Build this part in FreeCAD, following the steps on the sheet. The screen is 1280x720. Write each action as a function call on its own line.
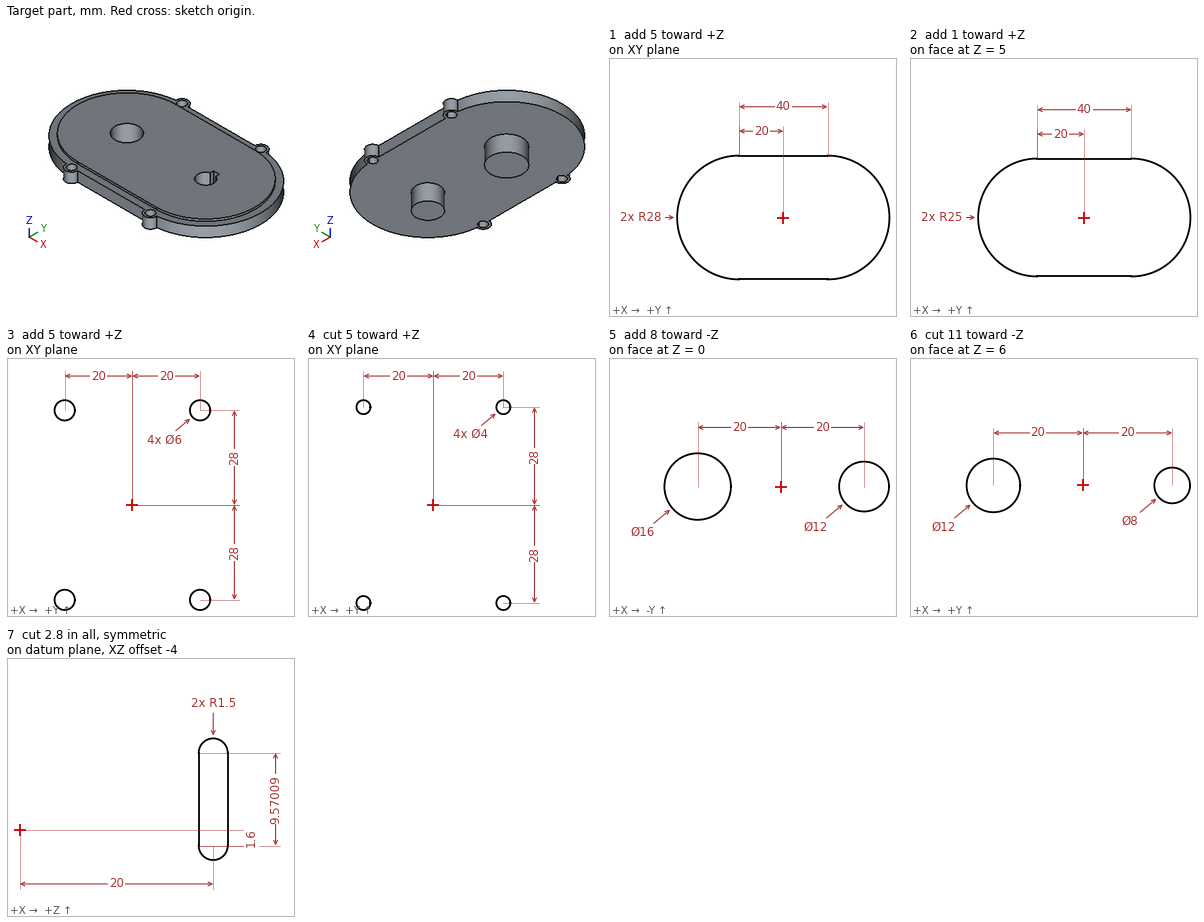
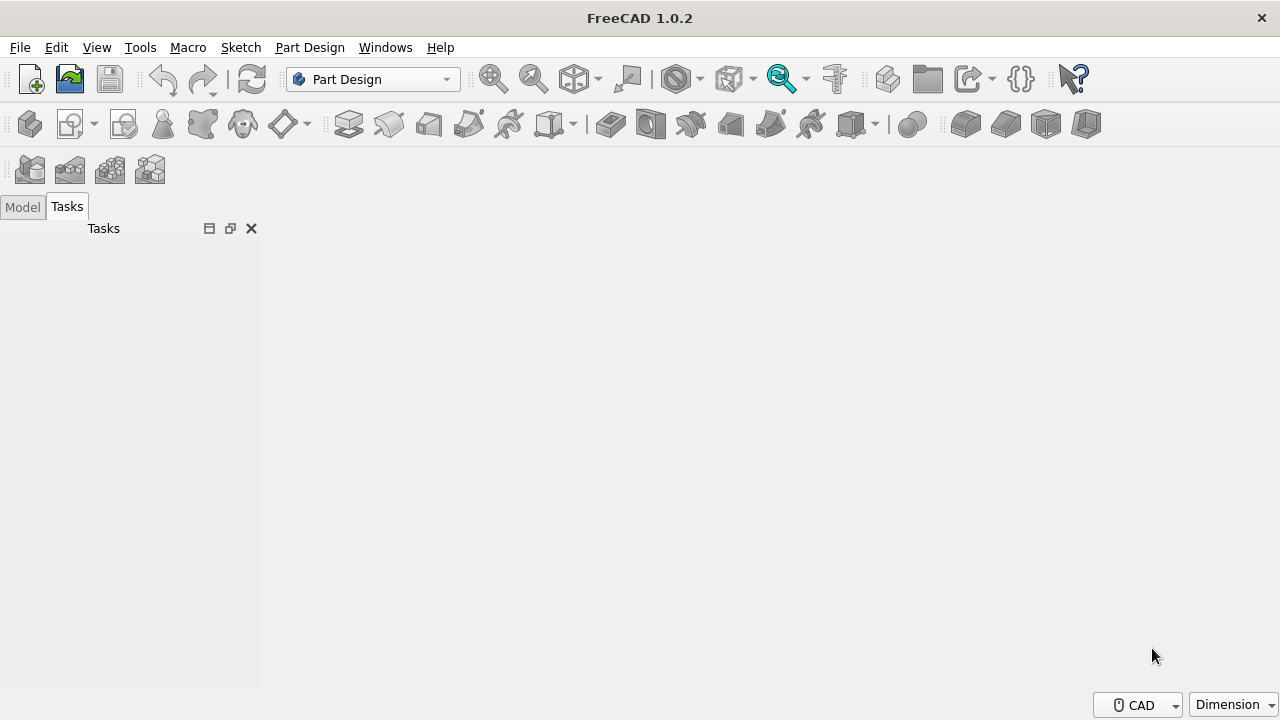
key(ctrl+n)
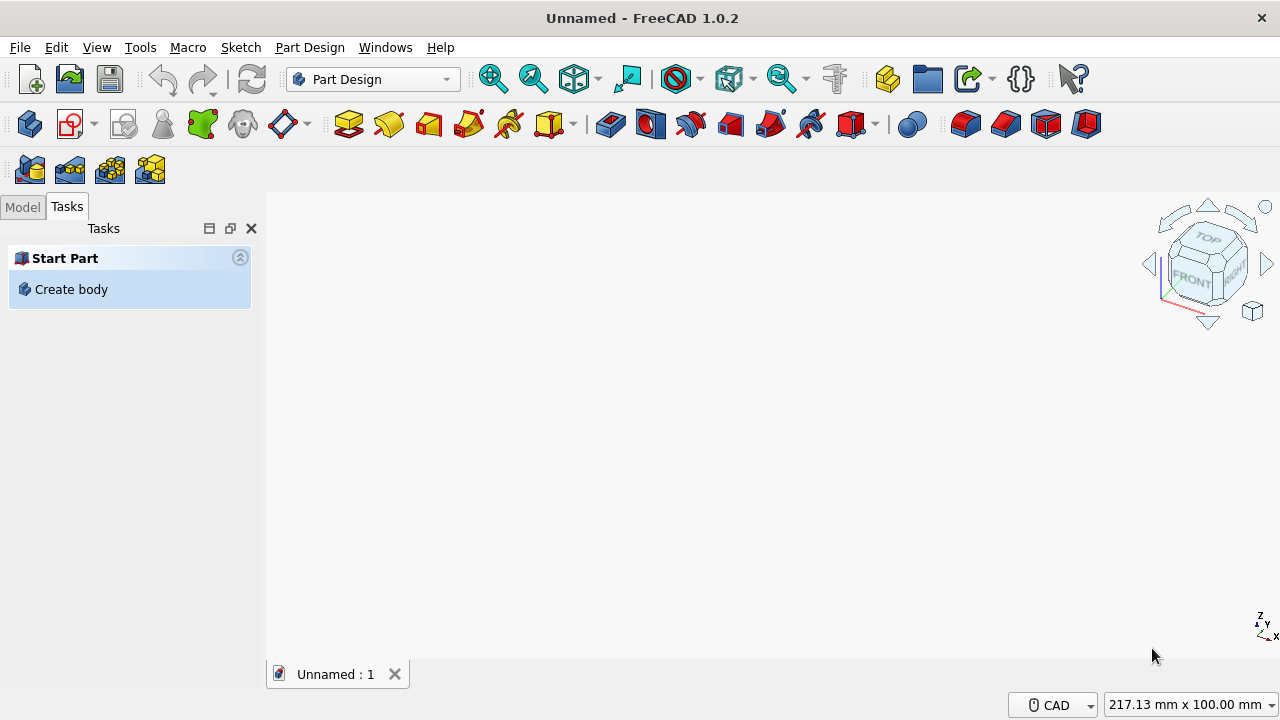
click(70, 124)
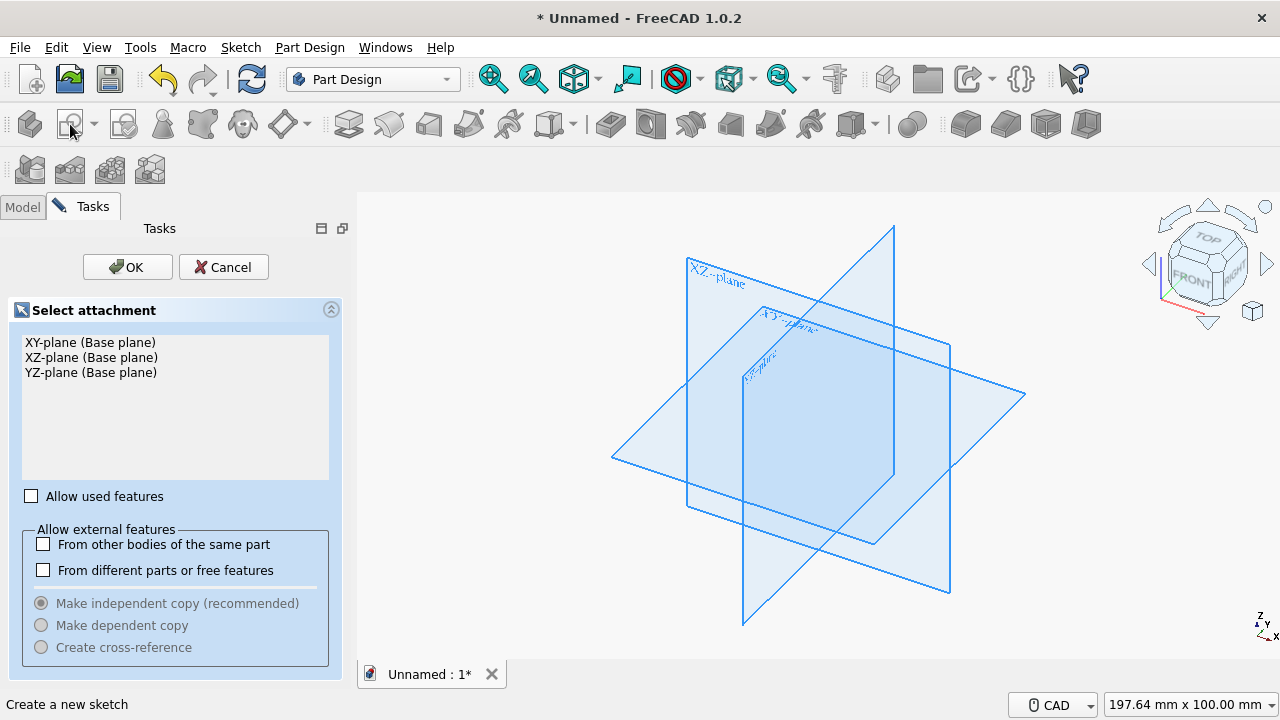
click(82, 342)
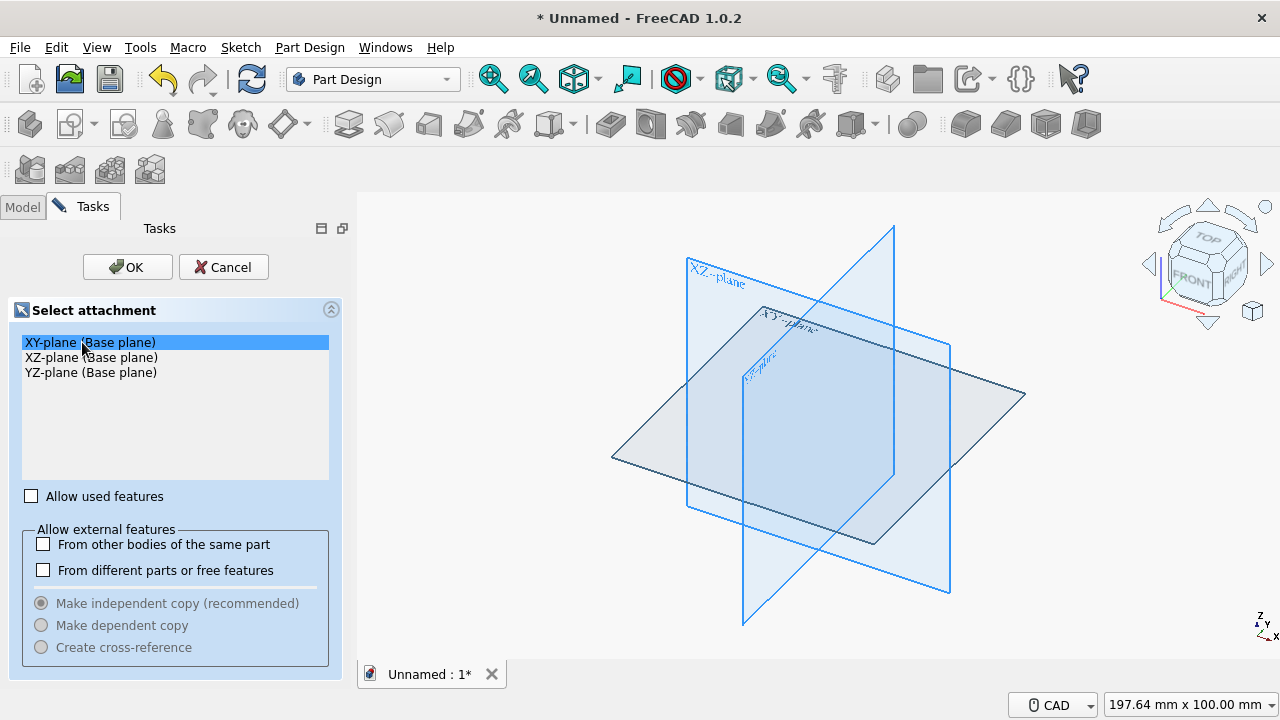
click(128, 267)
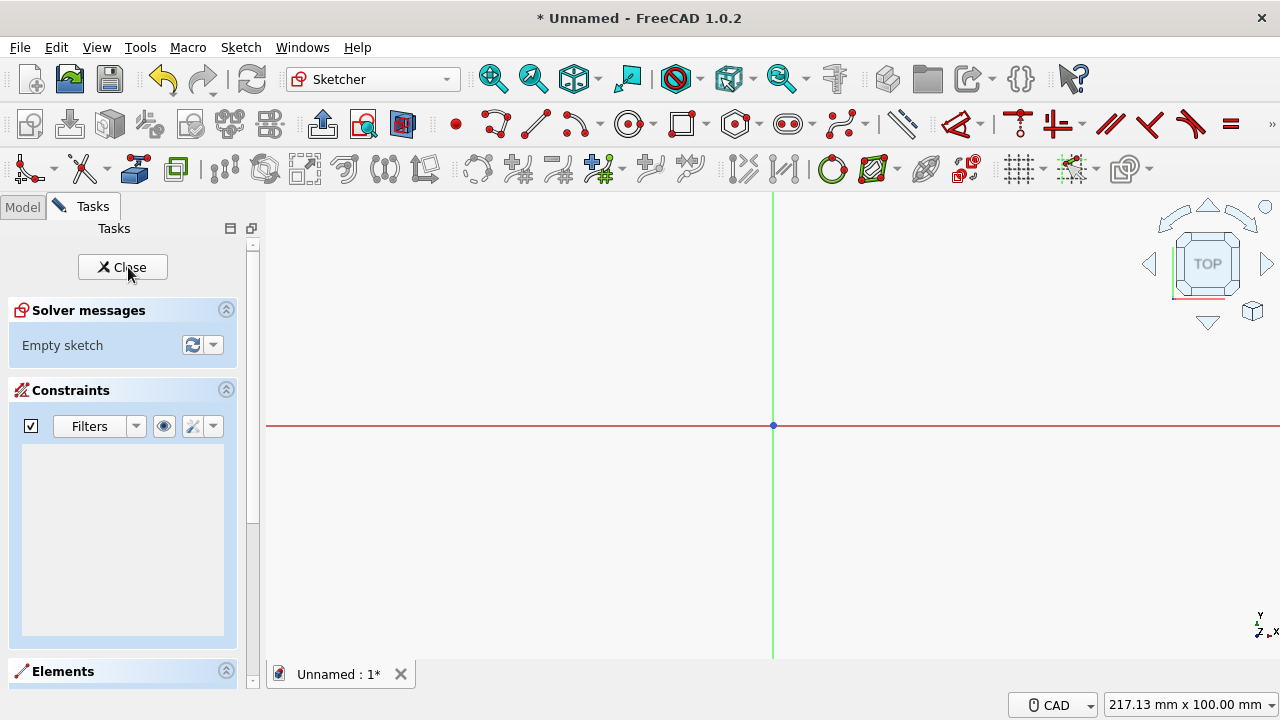
click(788, 124)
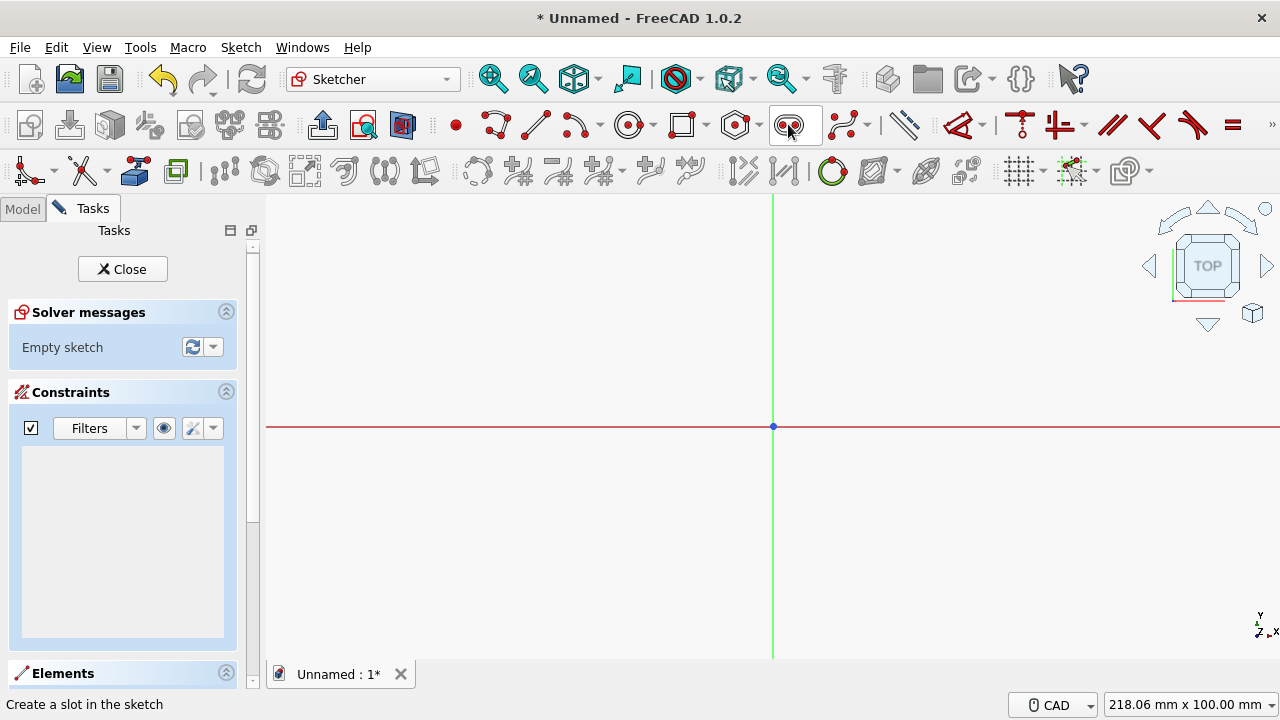
click(680, 426)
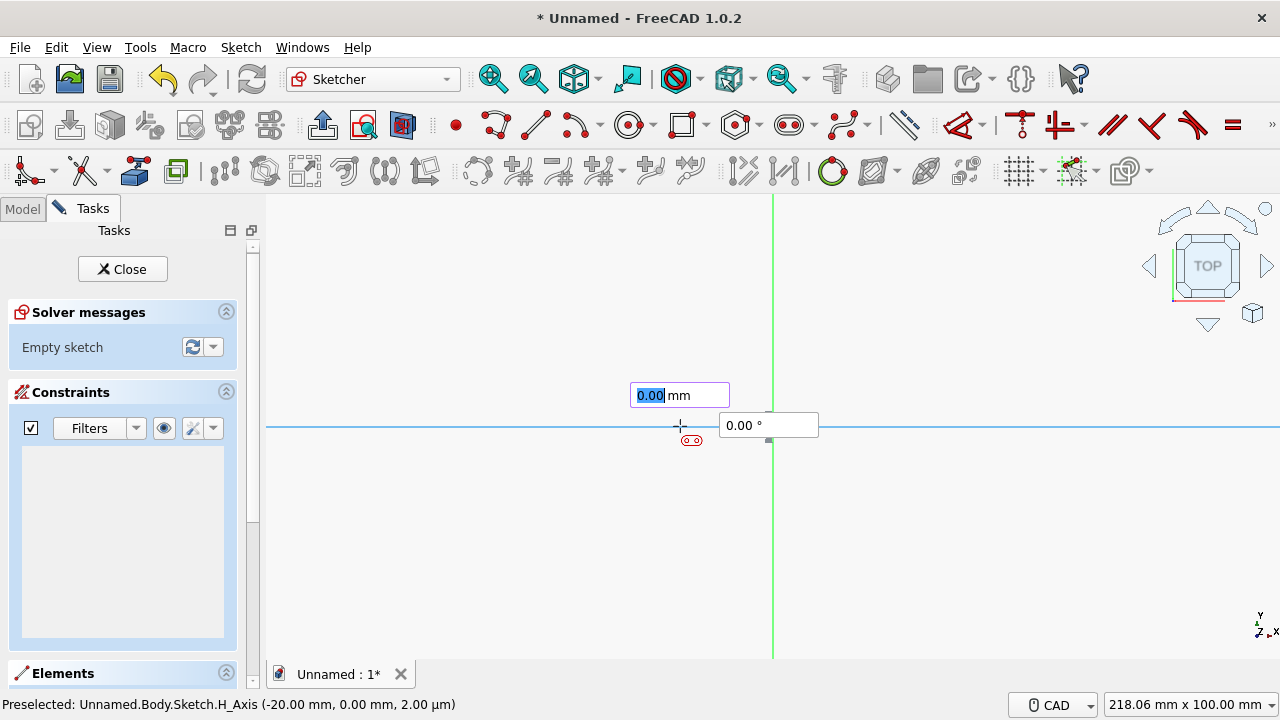
click(866, 418)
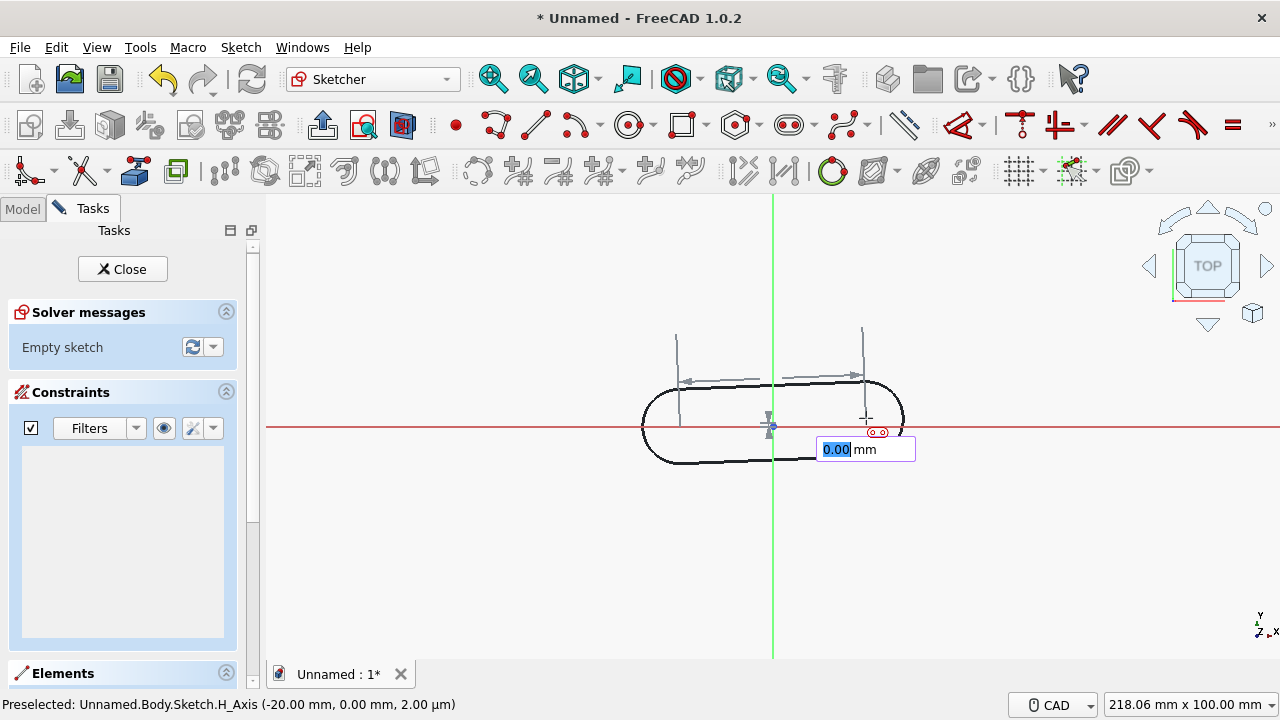
click(801, 296)
key(Escape)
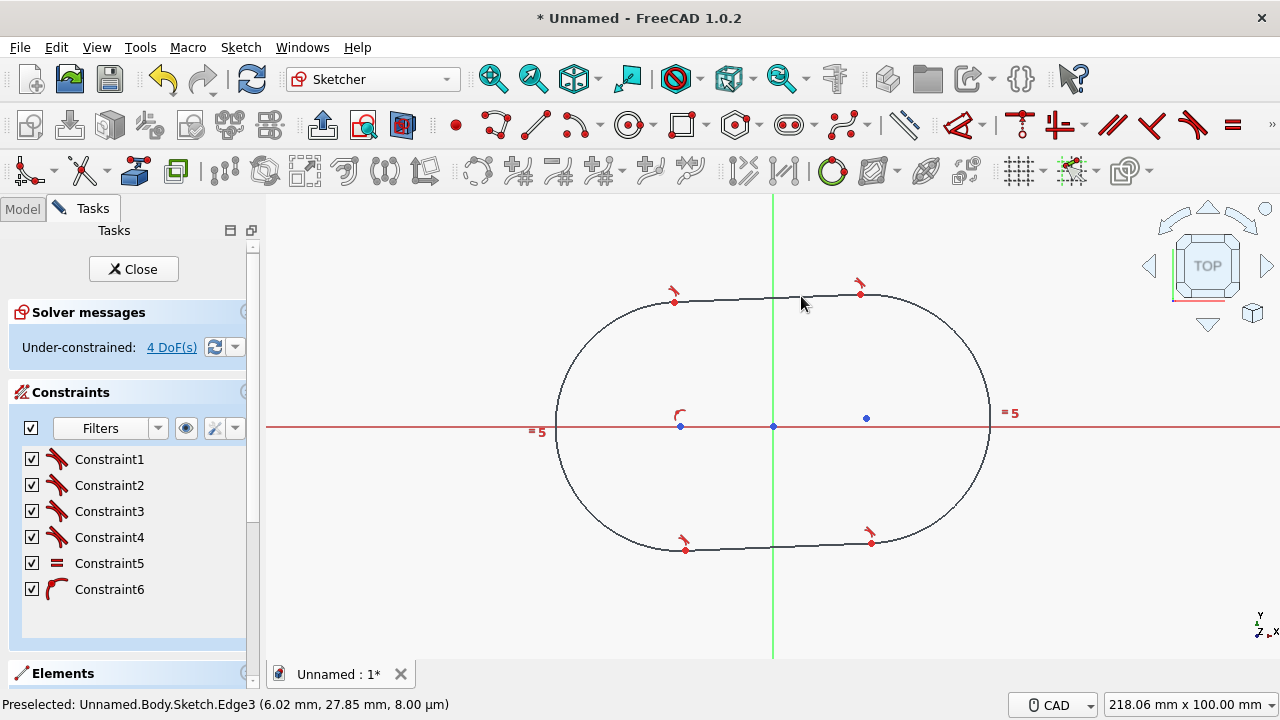
click(731, 300)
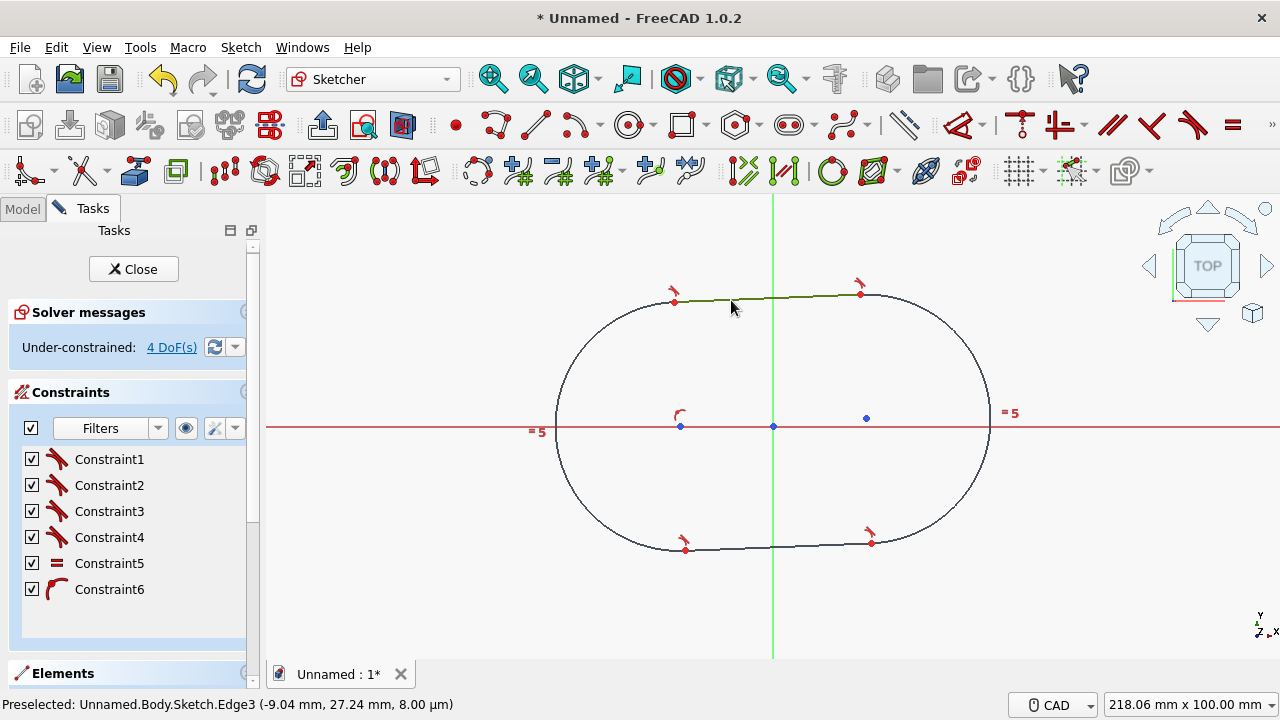
key(h)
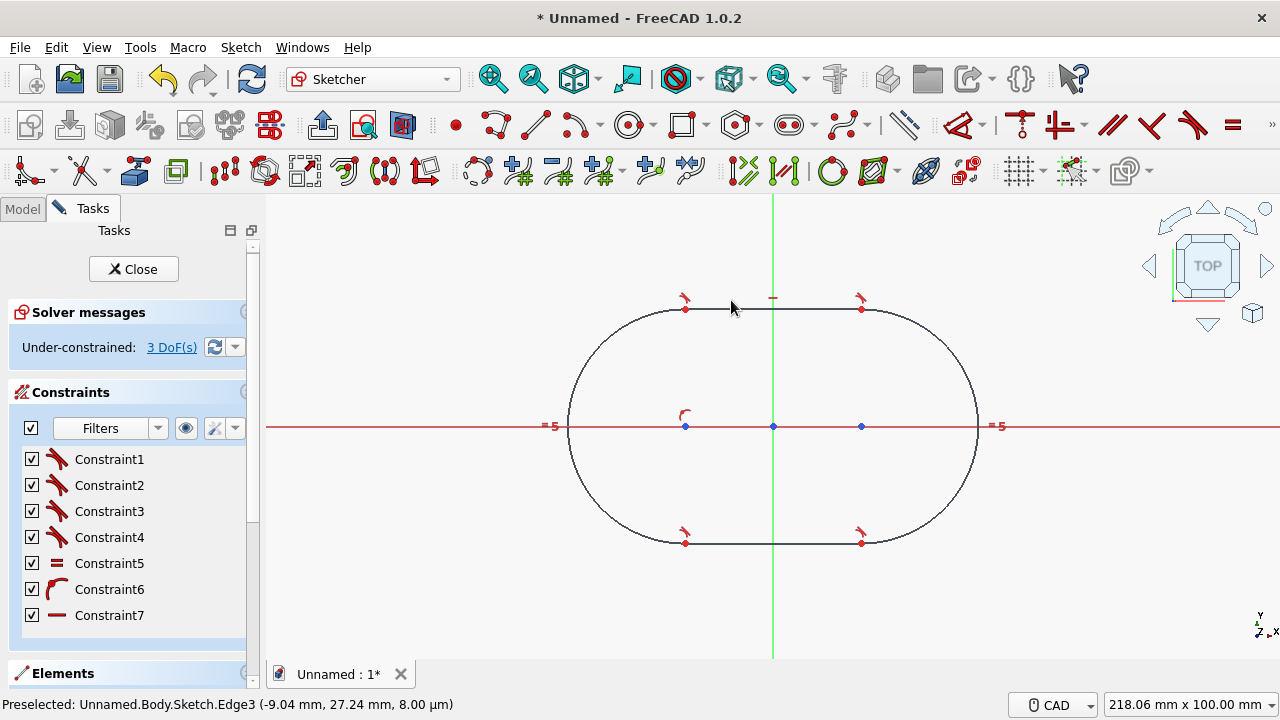
key(d)